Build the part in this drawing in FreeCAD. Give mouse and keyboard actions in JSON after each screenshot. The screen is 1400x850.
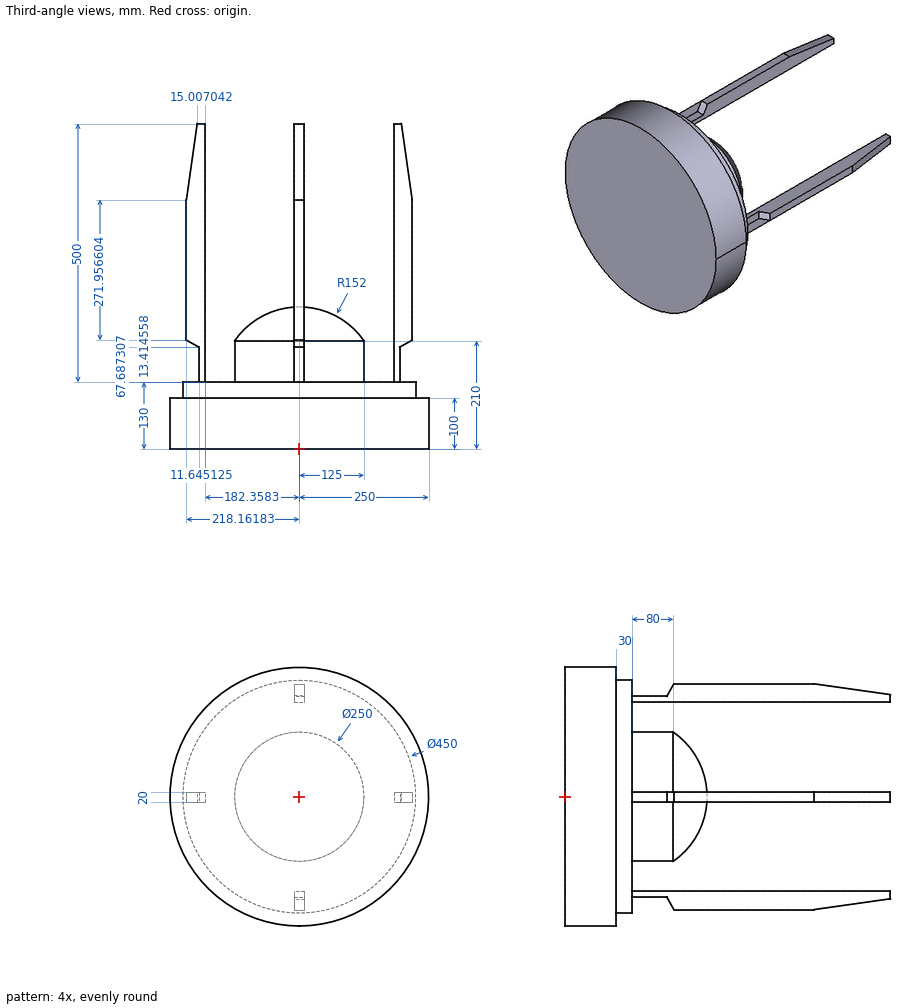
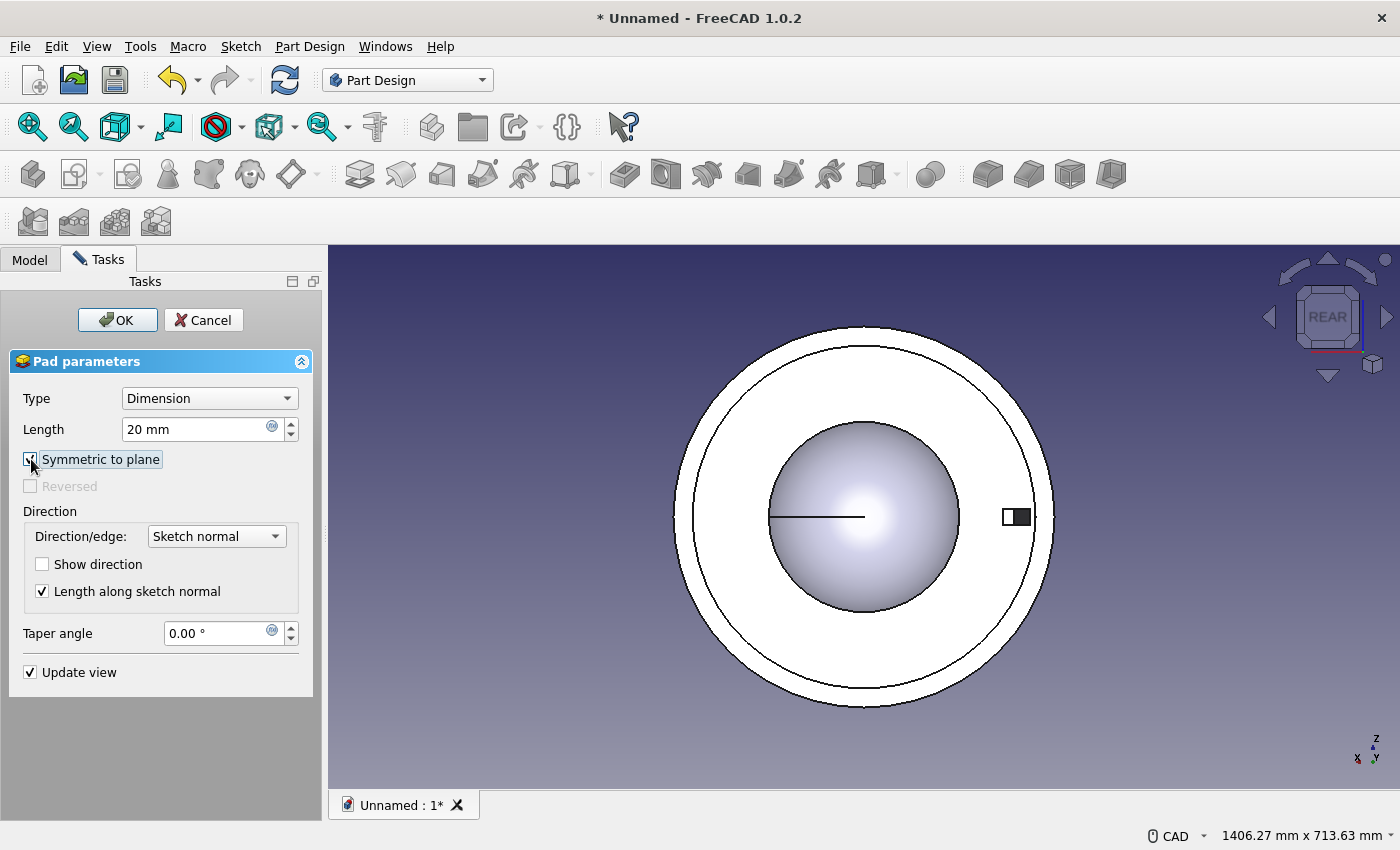
{"action": "left_click", "coordinate": [118, 320]}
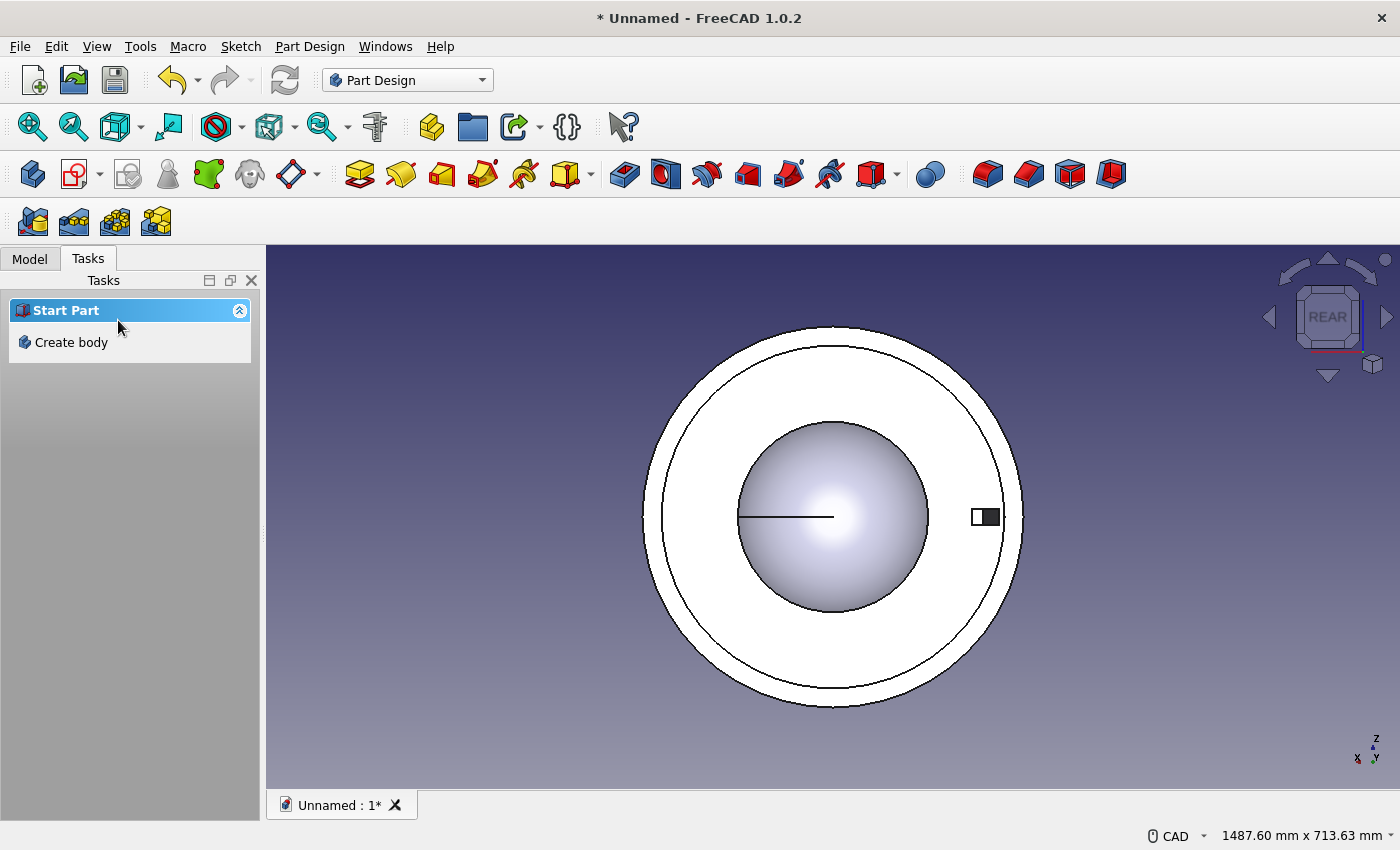
{"action": "left_click", "coordinate": [30, 258]}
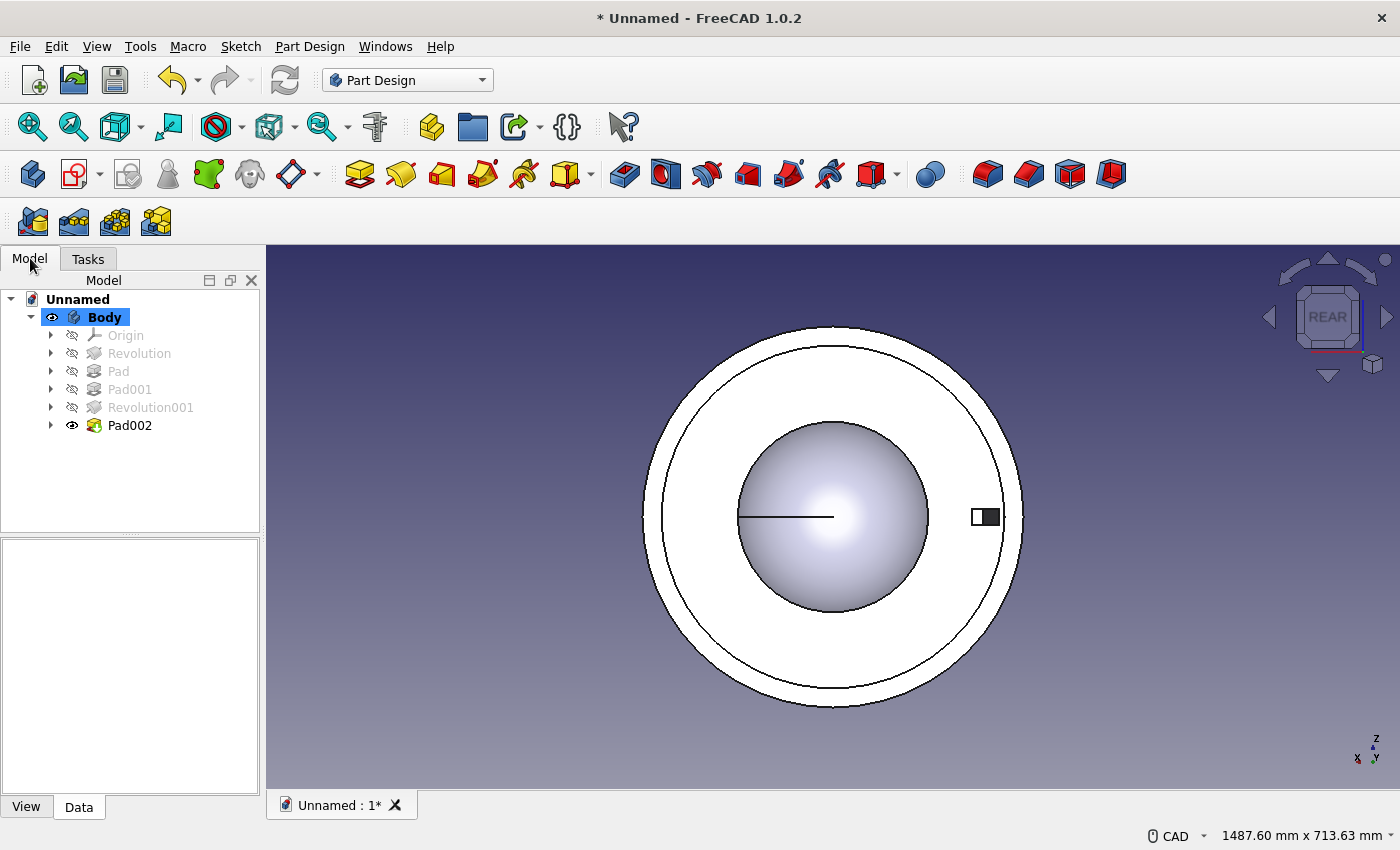
{"action": "left_click", "coordinate": [117, 425]}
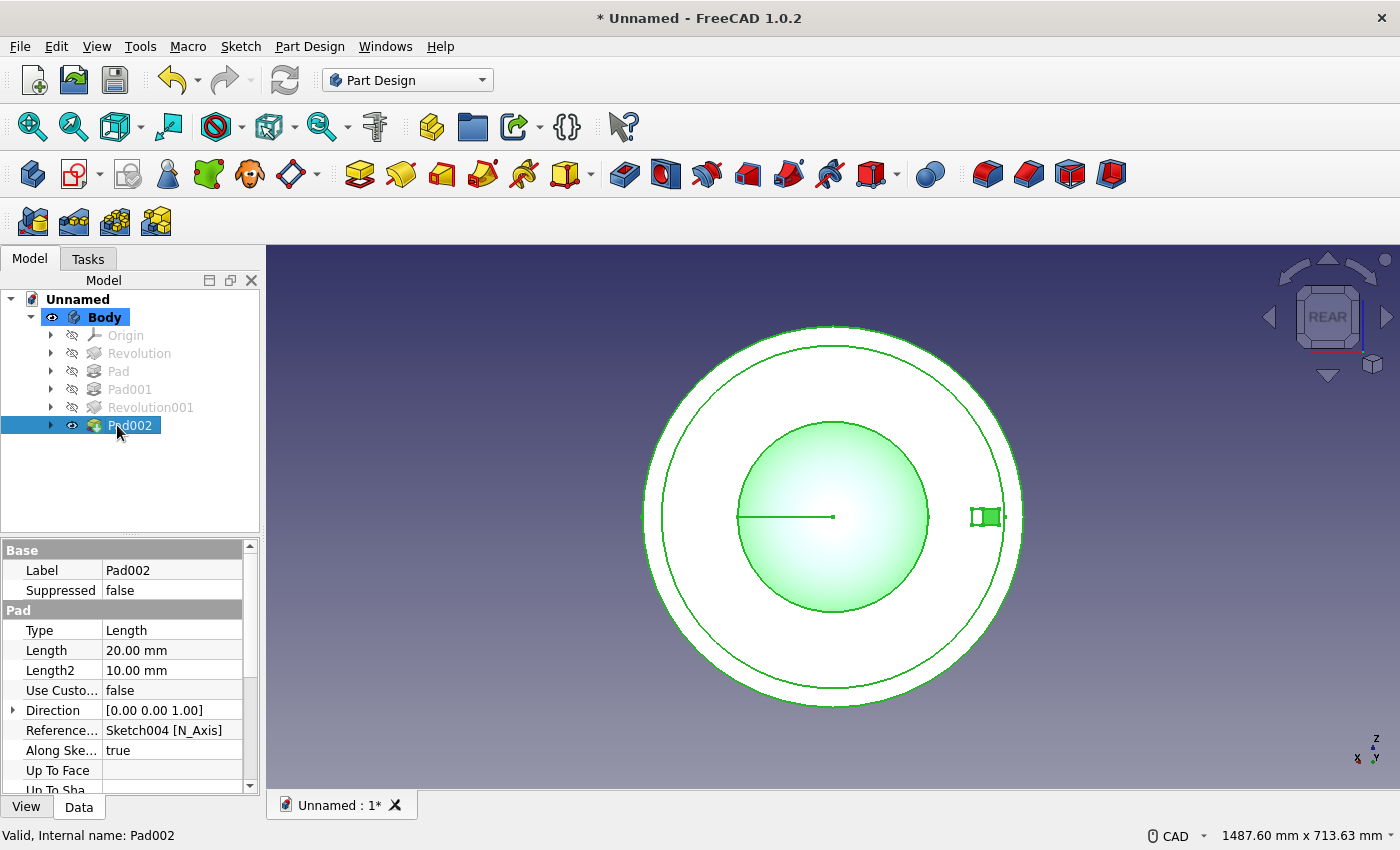
{"action": "left_click", "coordinate": [115, 222]}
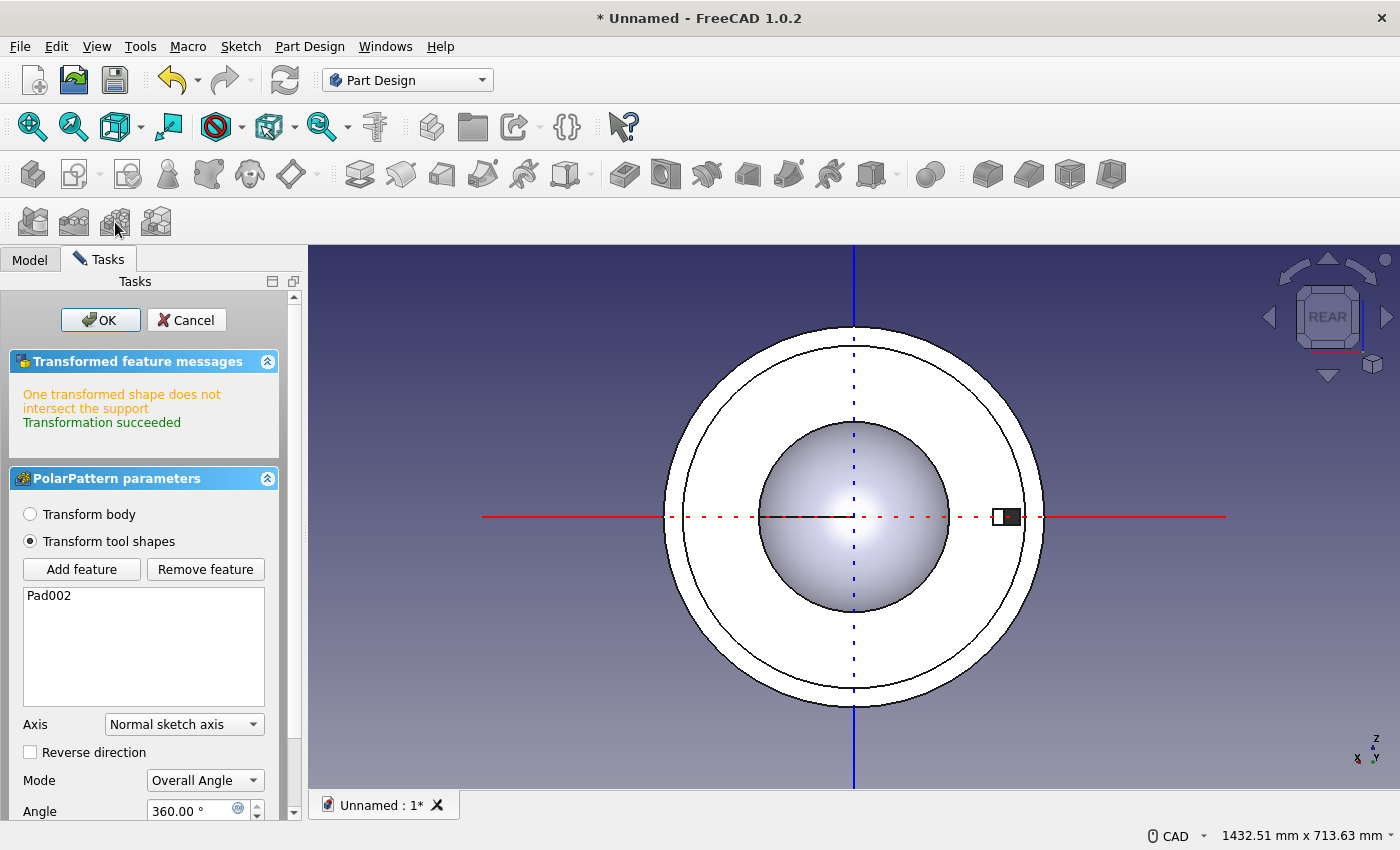
{"action": "left_click", "coordinate": [185, 724]}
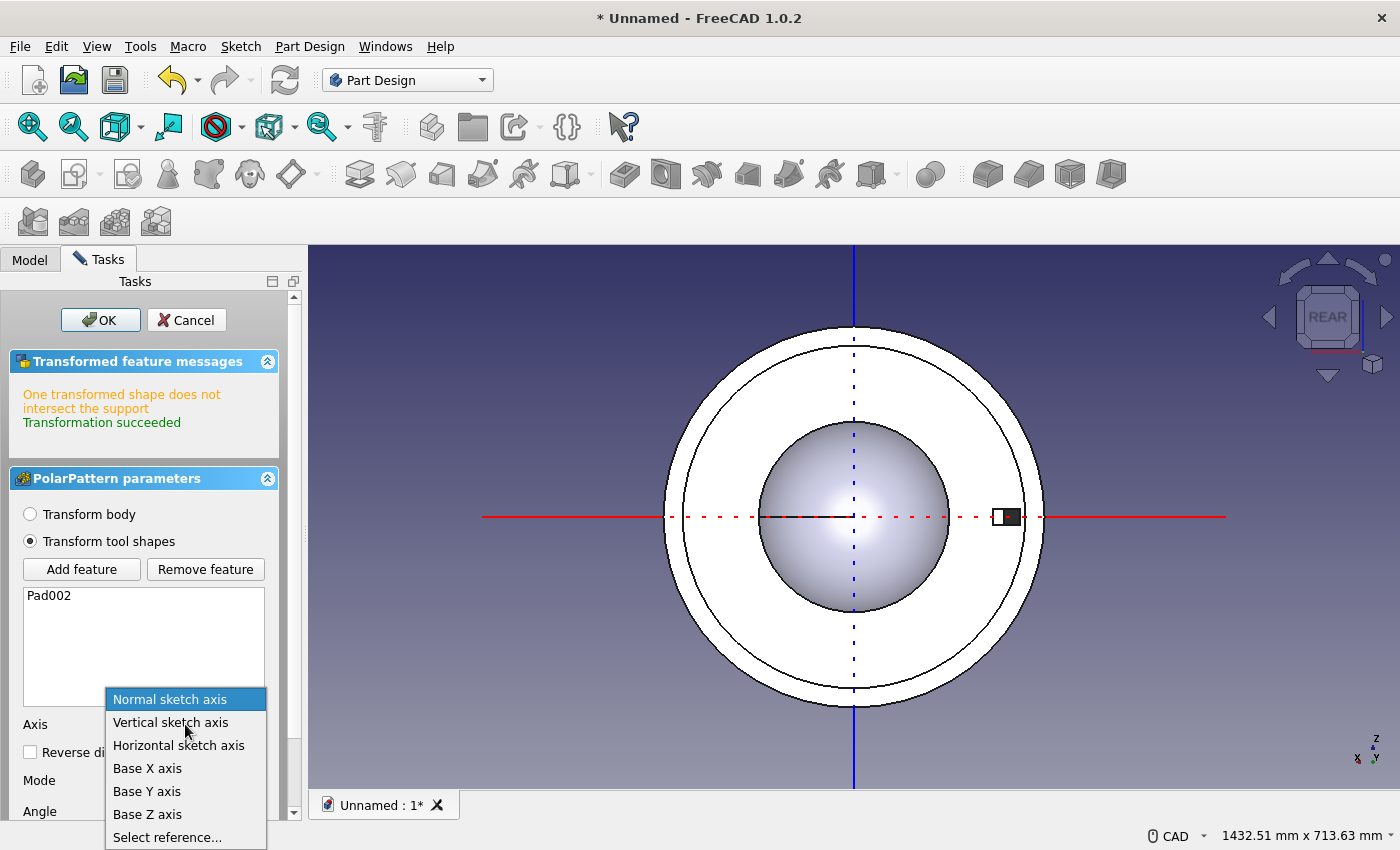
{"action": "left_click", "coordinate": [184, 792]}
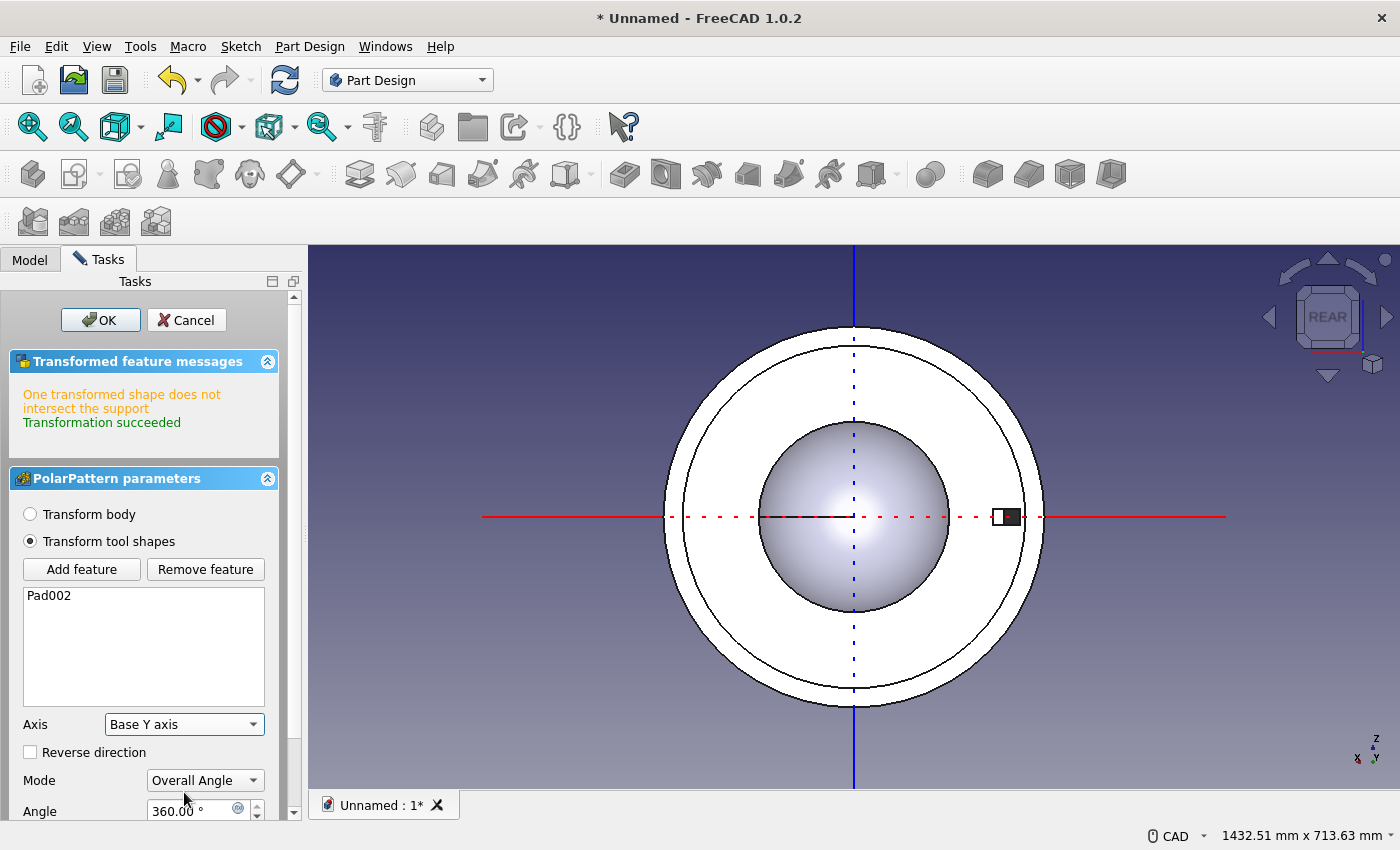
{"action": "scroll", "coordinate": [294, 556], "scroll_direction": "down", "scroll_amount": 2}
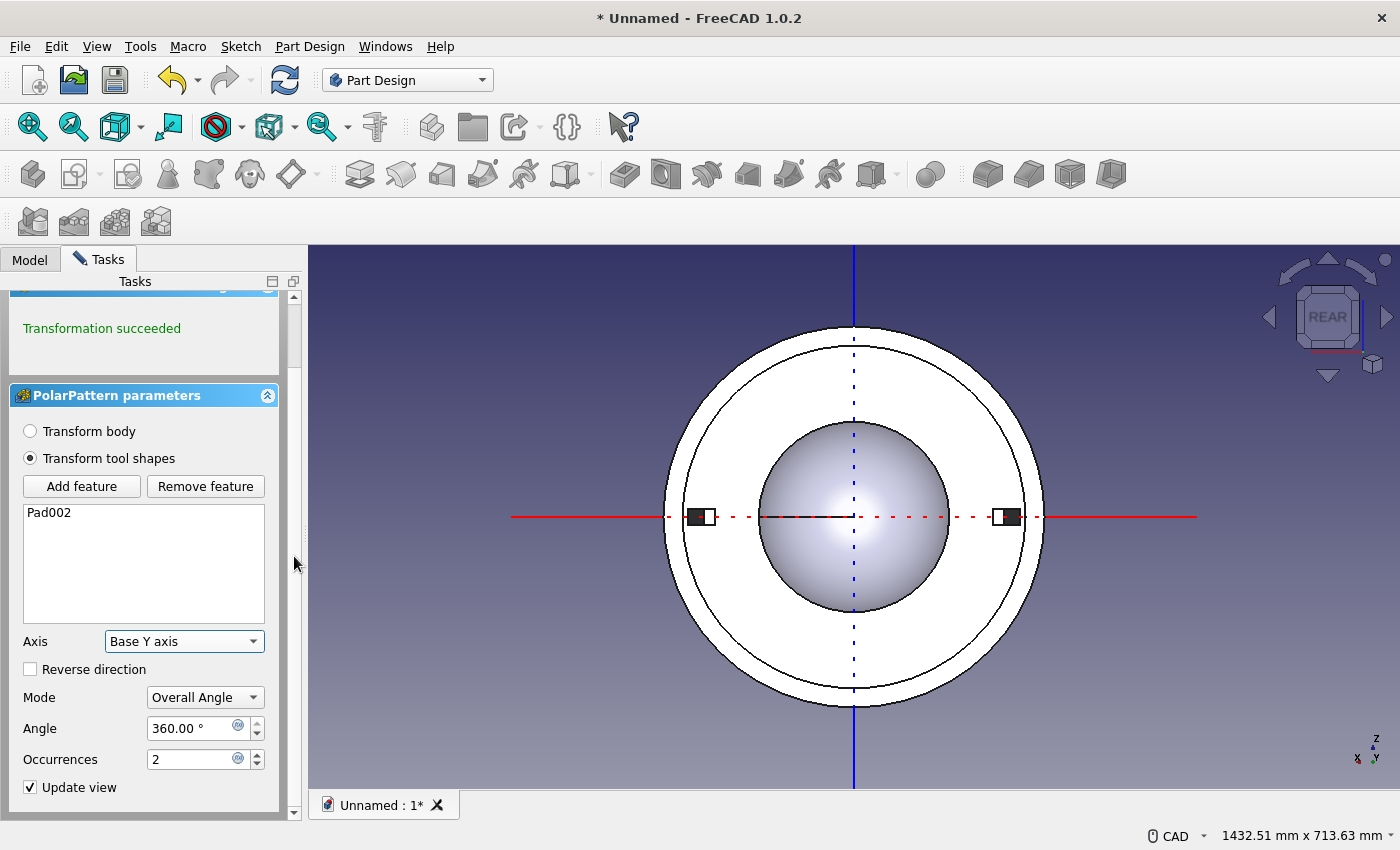
{"action": "triple_click", "coordinate": [199, 760]}